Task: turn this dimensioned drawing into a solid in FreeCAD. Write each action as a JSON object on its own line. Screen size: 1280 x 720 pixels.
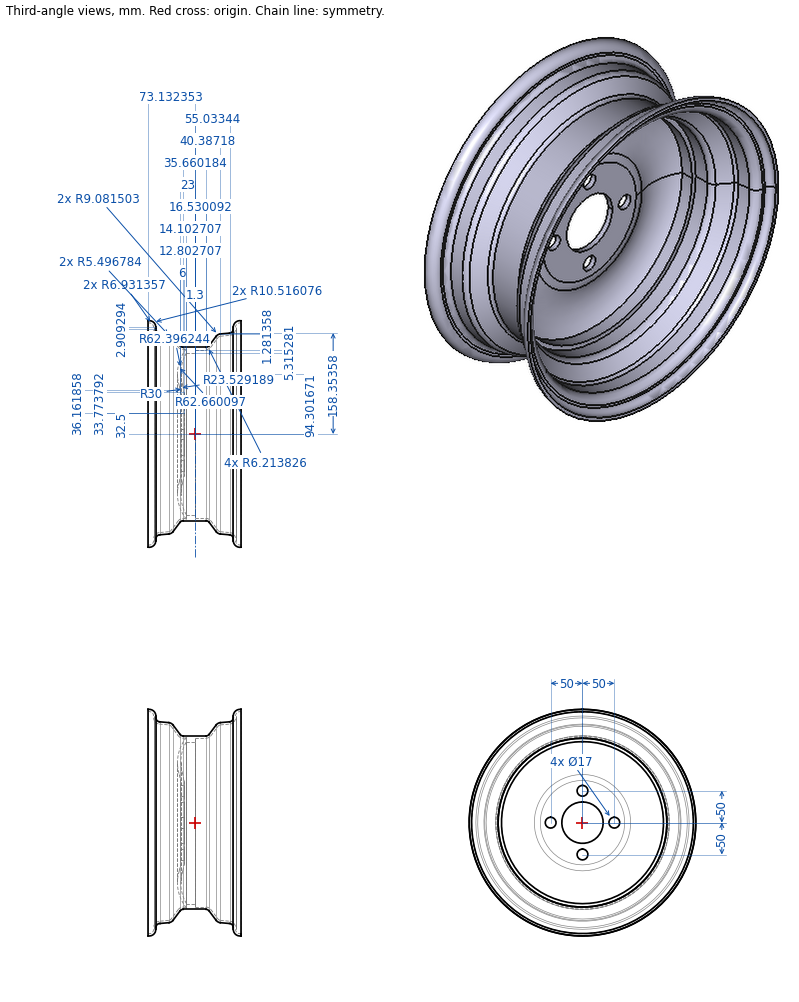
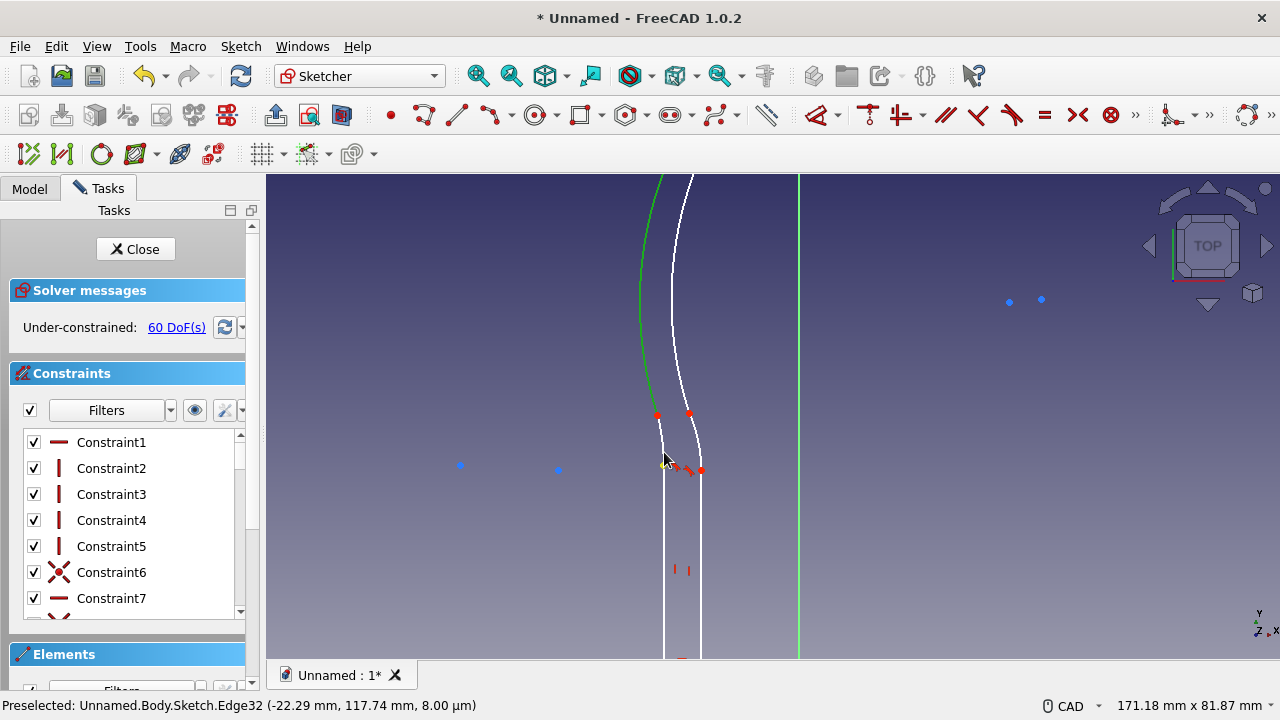
{"action": "left_click", "coordinate": [663, 450]}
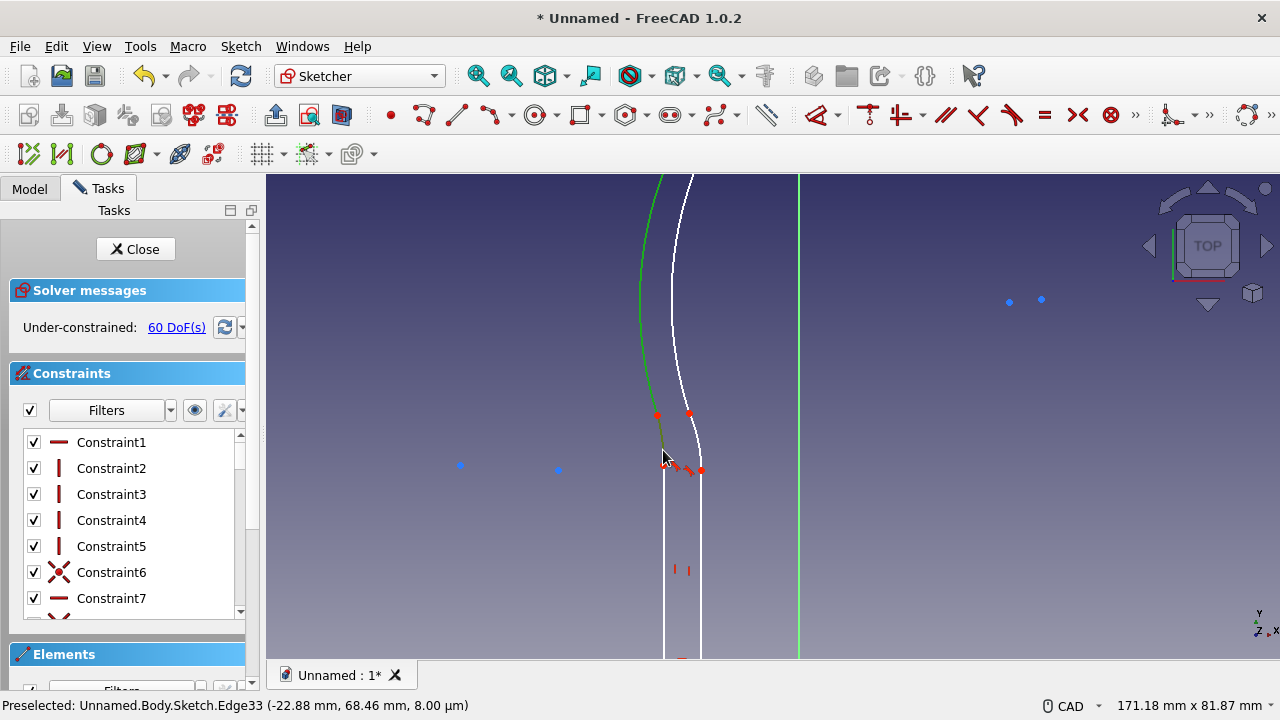
{"action": "left_click", "coordinate": [1012, 116]}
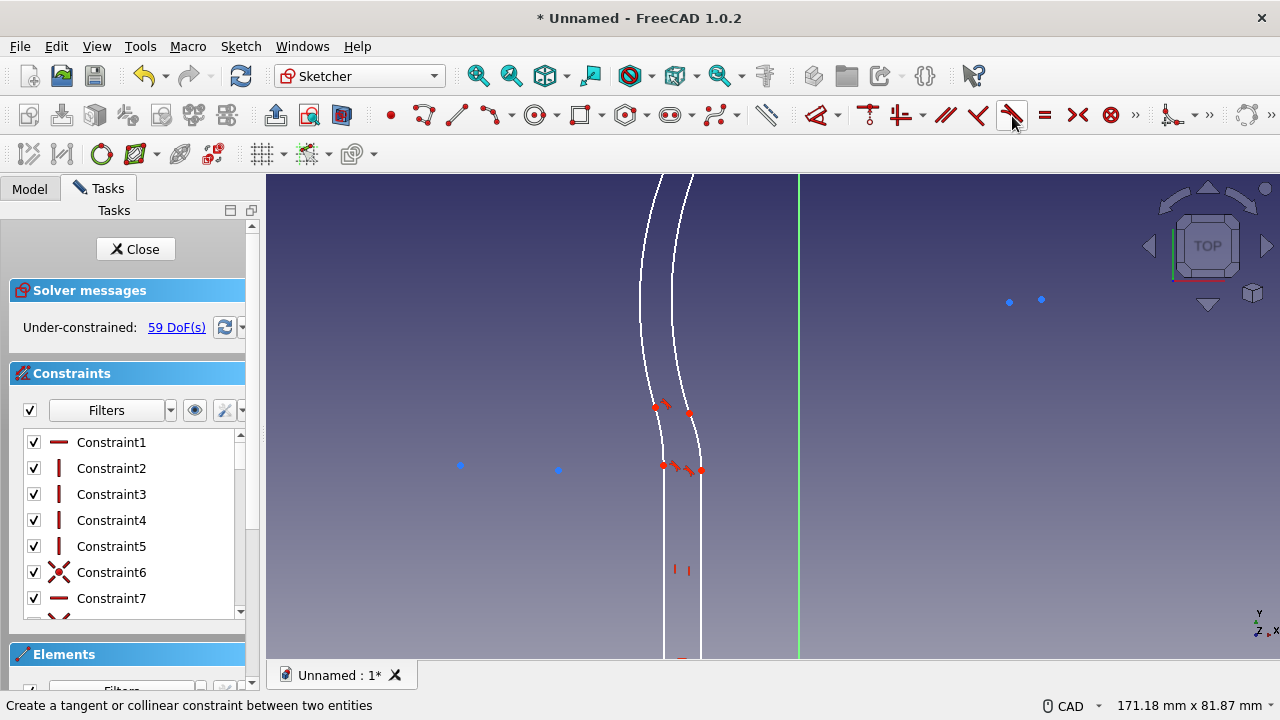
{"action": "left_click", "coordinate": [700, 453]}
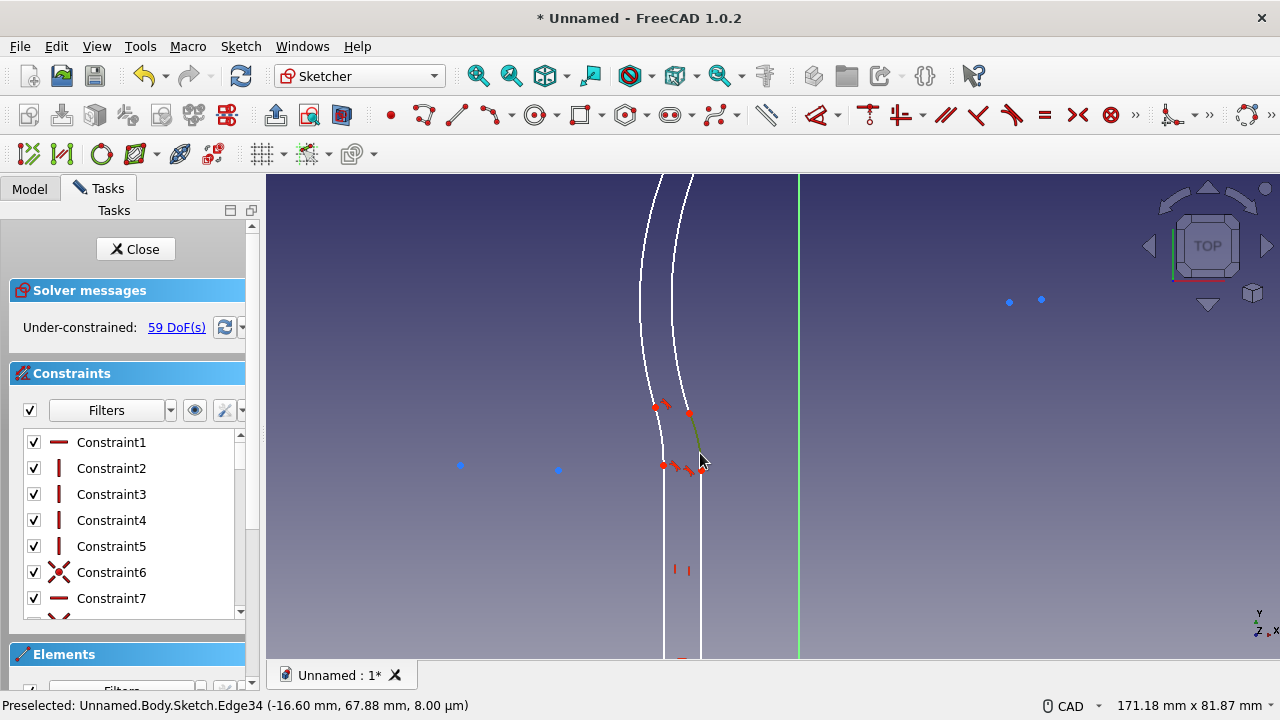
{"action": "left_click", "coordinate": [672, 321]}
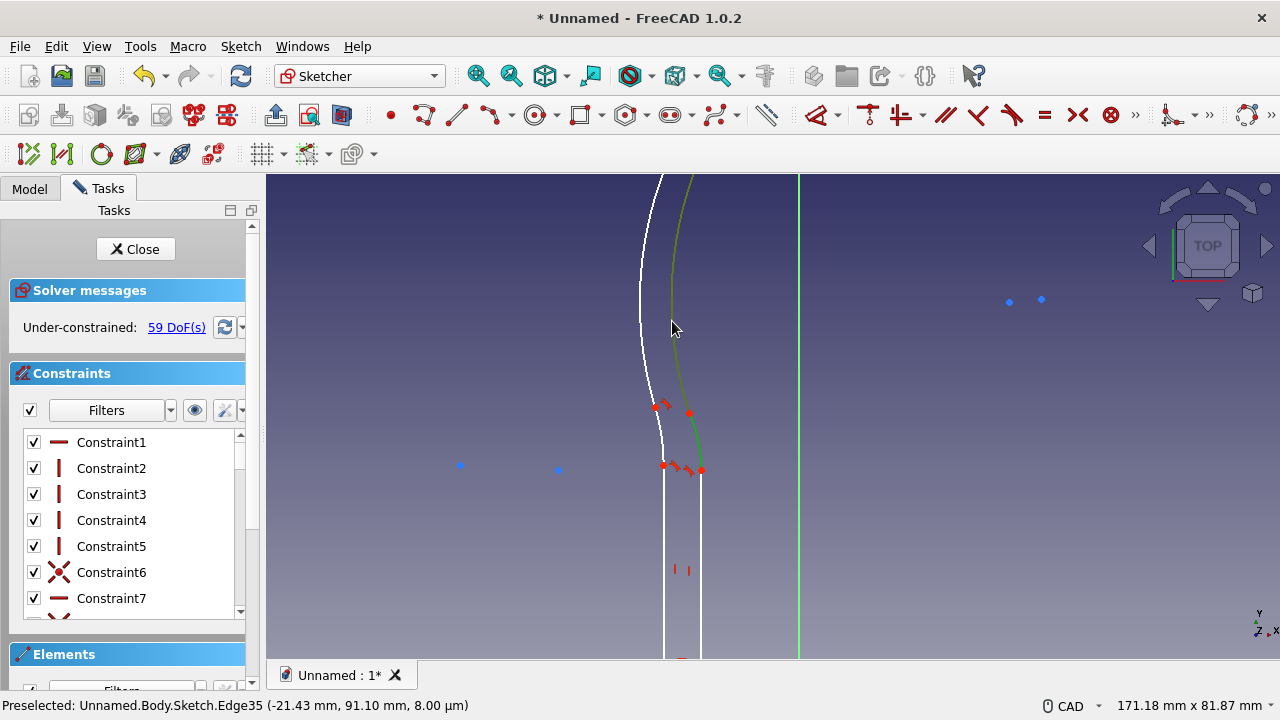
{"action": "key", "text": "t"}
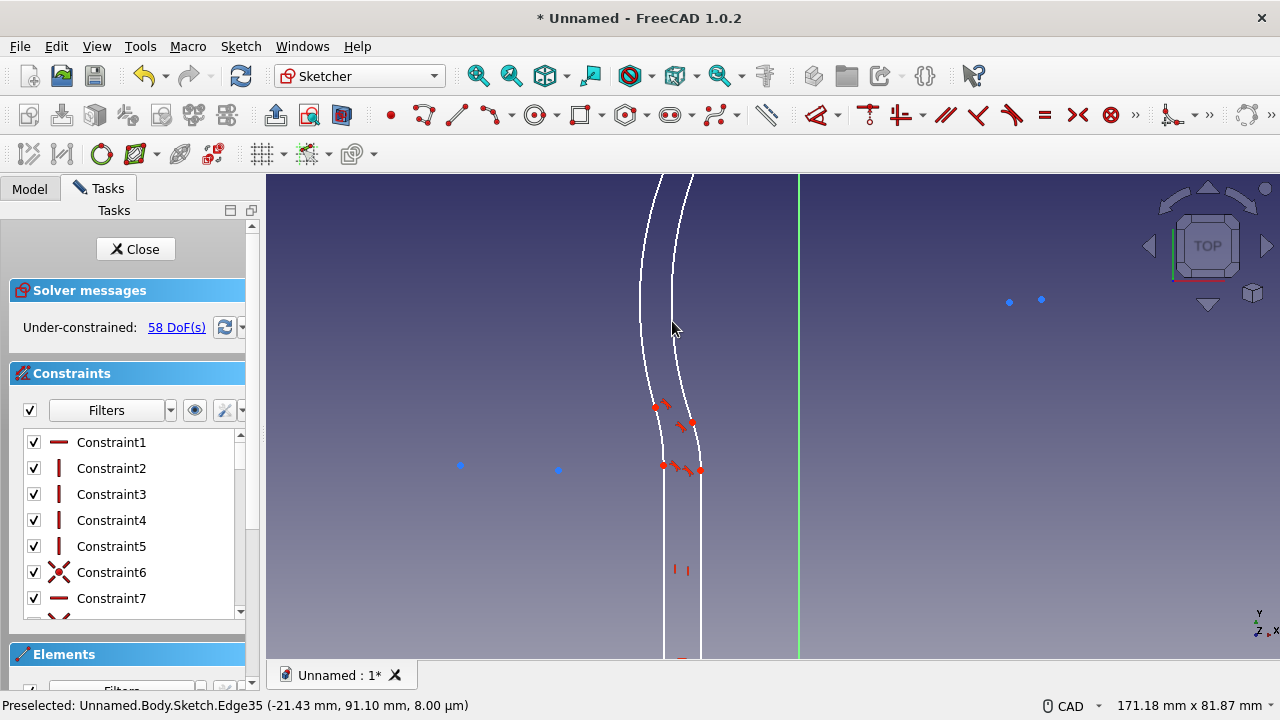
{"action": "scroll", "coordinate": [664, 452], "scroll_direction": "down", "scroll_amount": 6}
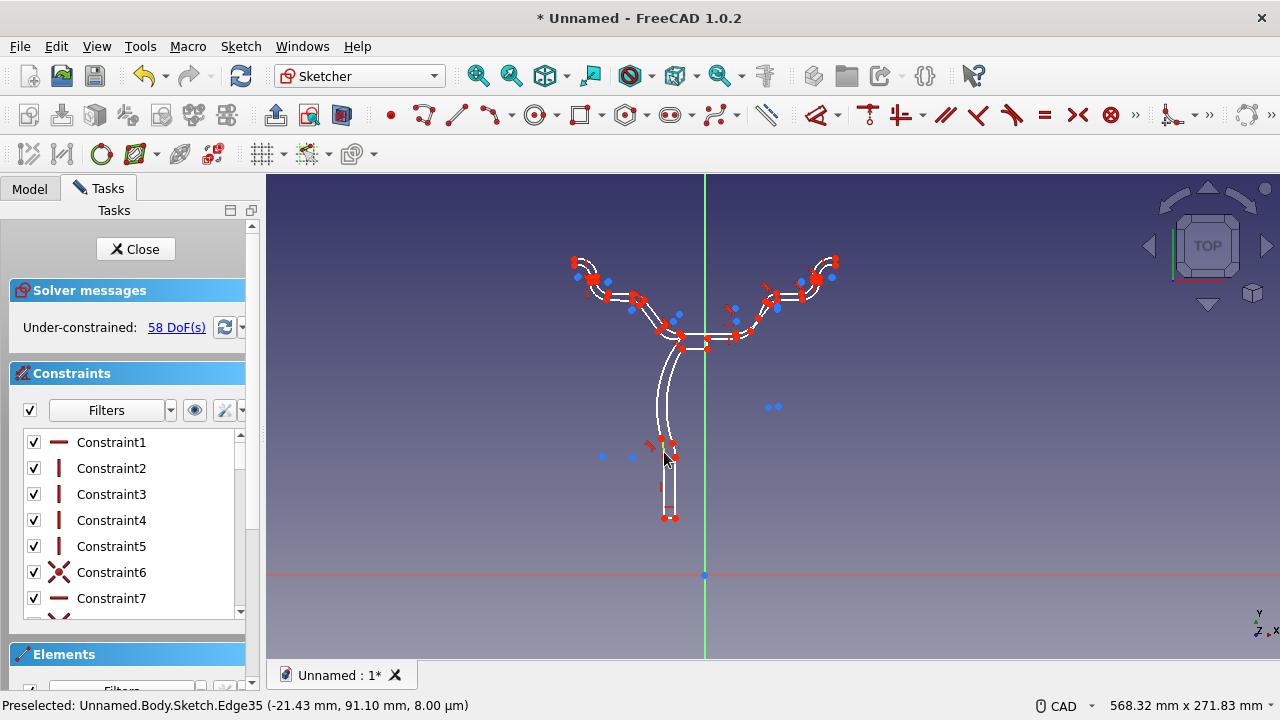
{"action": "scroll", "coordinate": [594, 268], "scroll_direction": "up", "scroll_amount": 4}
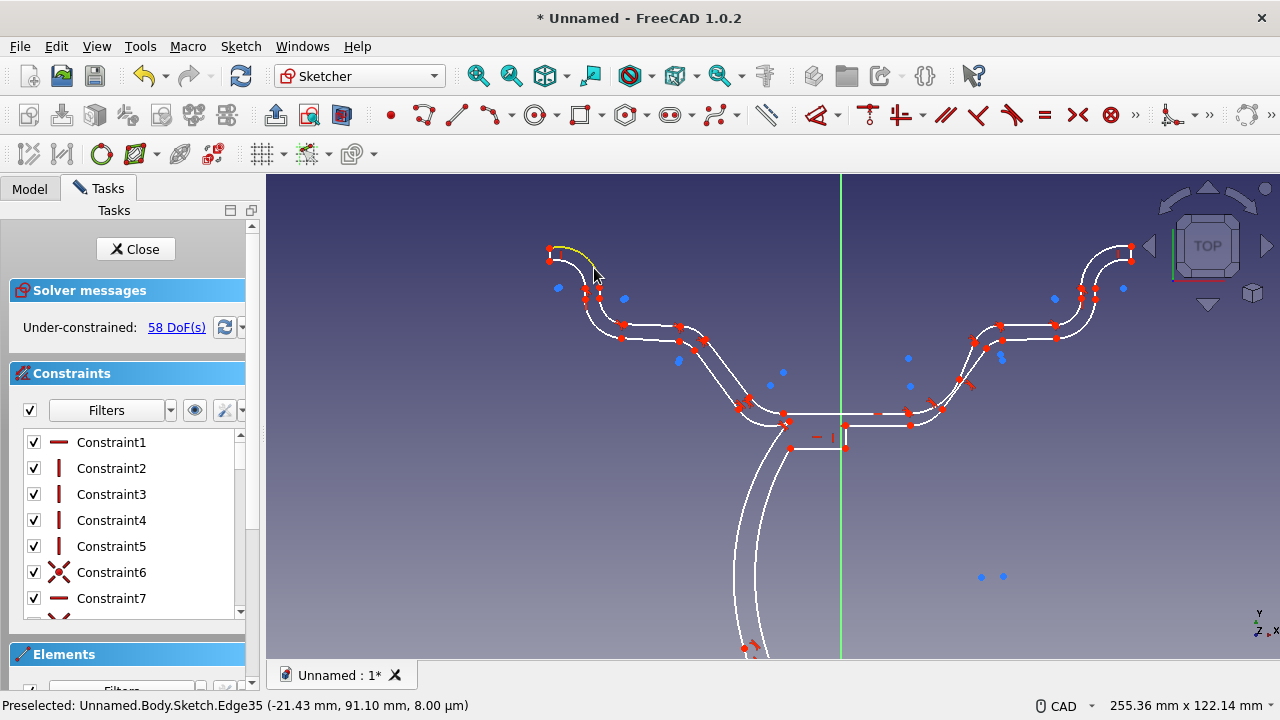
{"action": "left_click", "coordinate": [594, 267]}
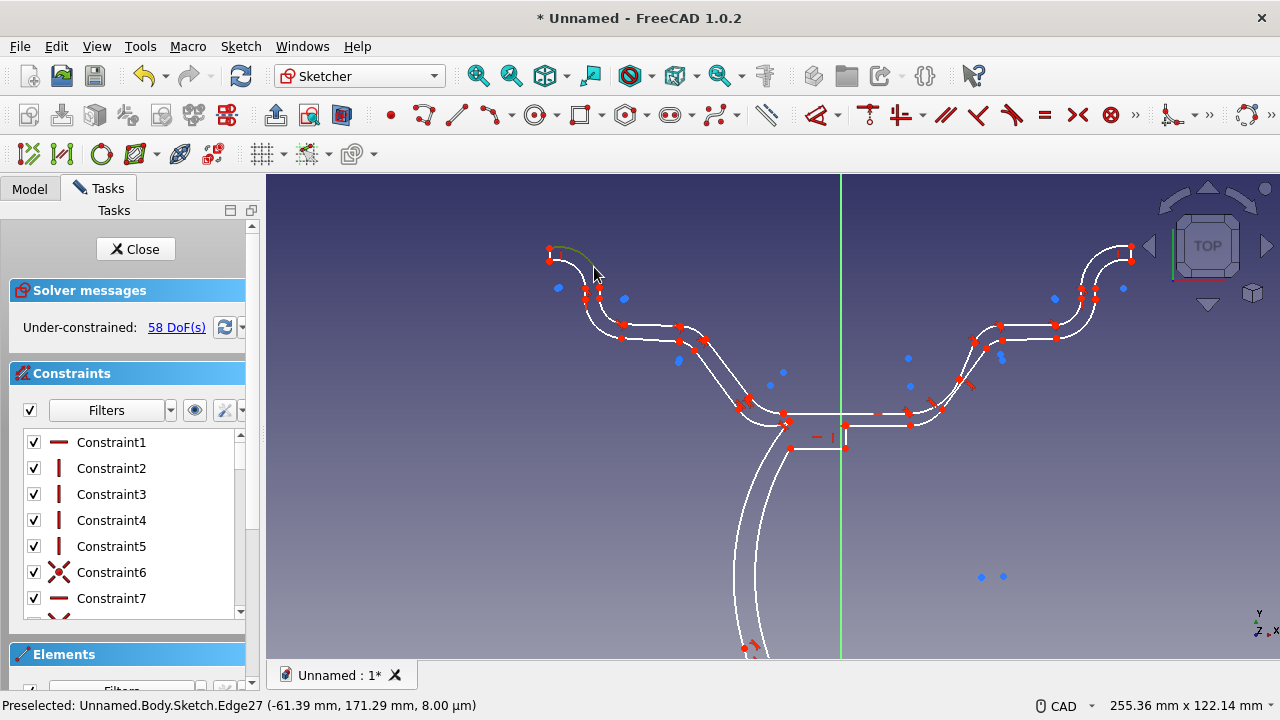
{"action": "left_click", "coordinate": [581, 273]}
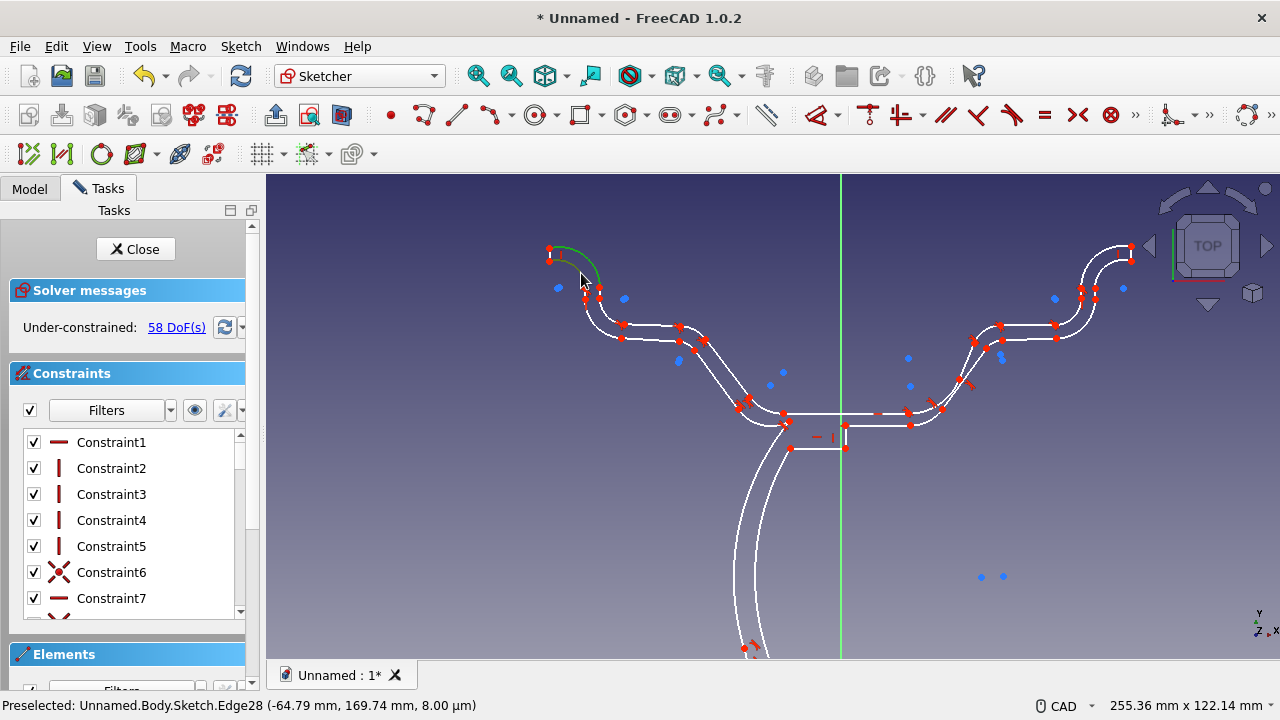
{"action": "key", "text": "c"}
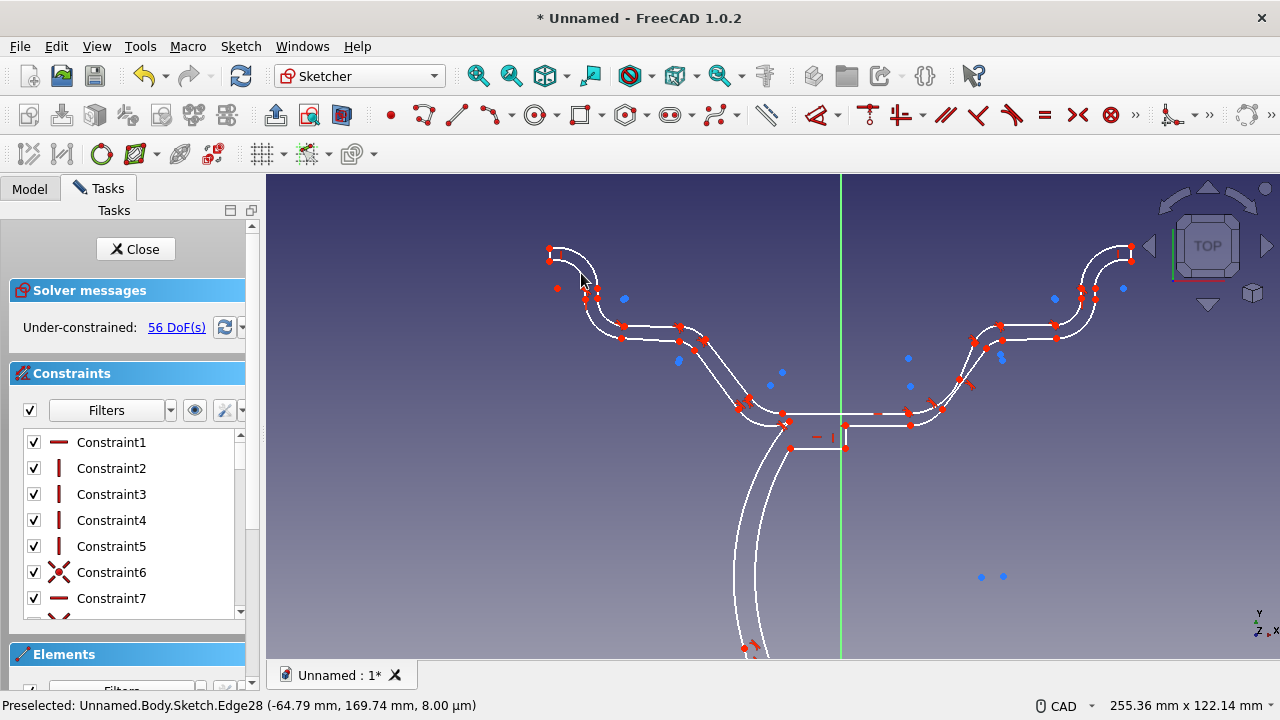
{"action": "left_click", "coordinate": [612, 323]}